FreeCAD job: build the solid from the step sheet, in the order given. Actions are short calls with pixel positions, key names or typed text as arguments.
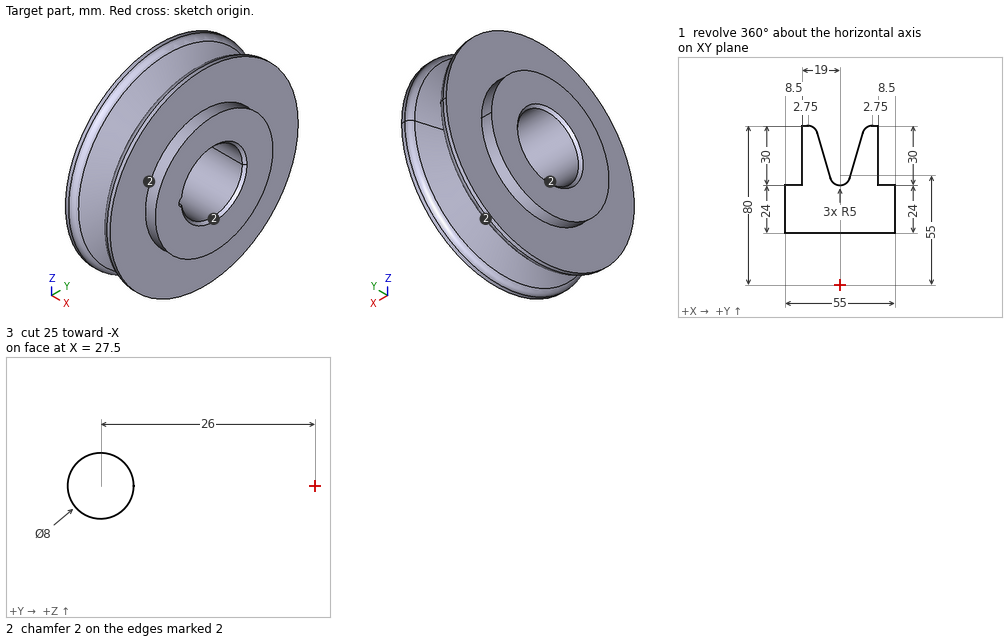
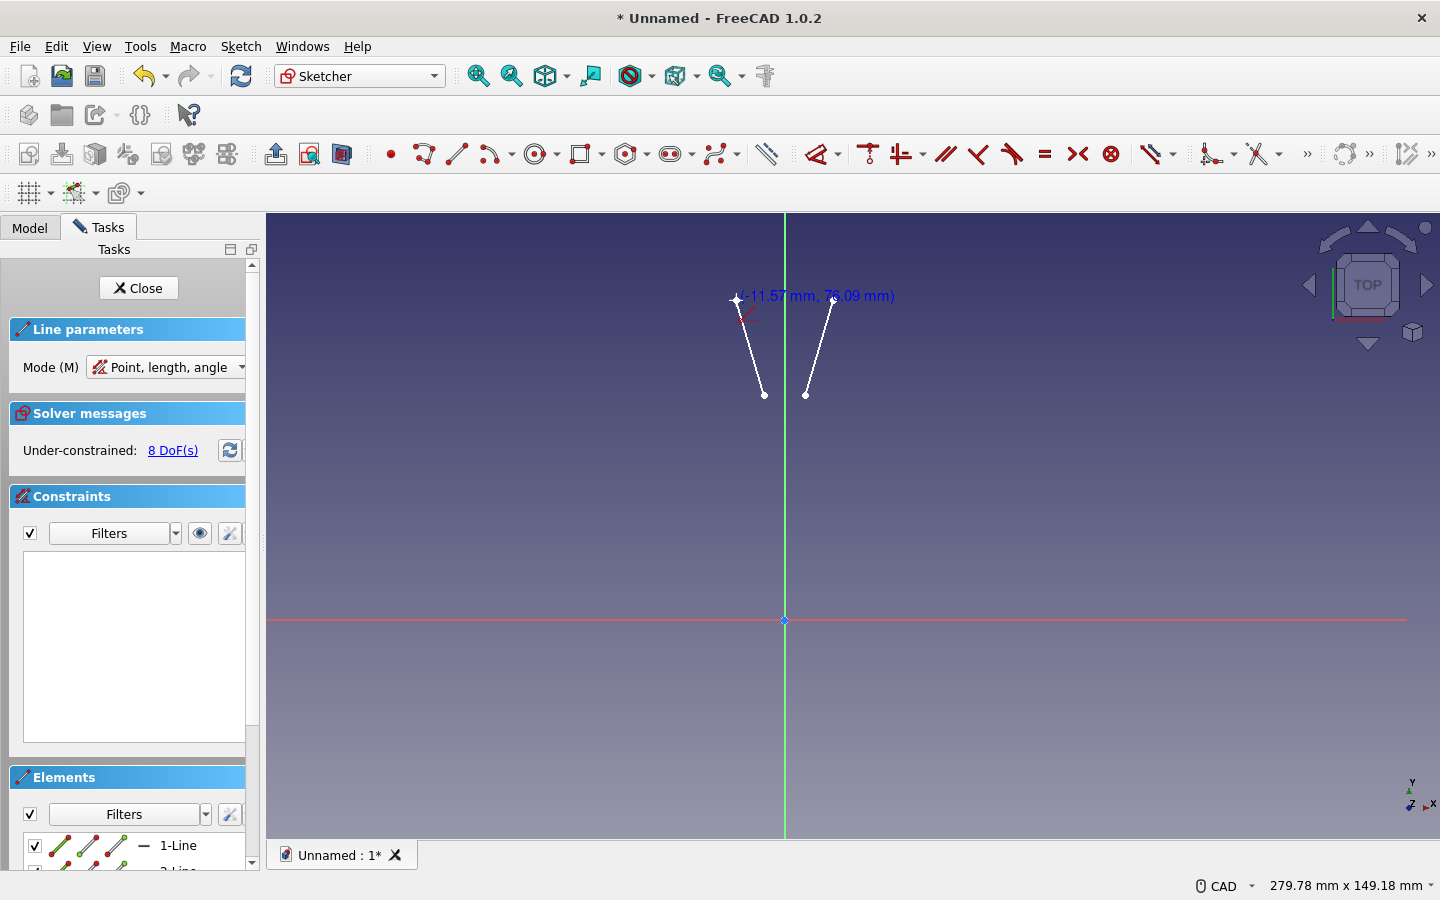
key(g)
key(m)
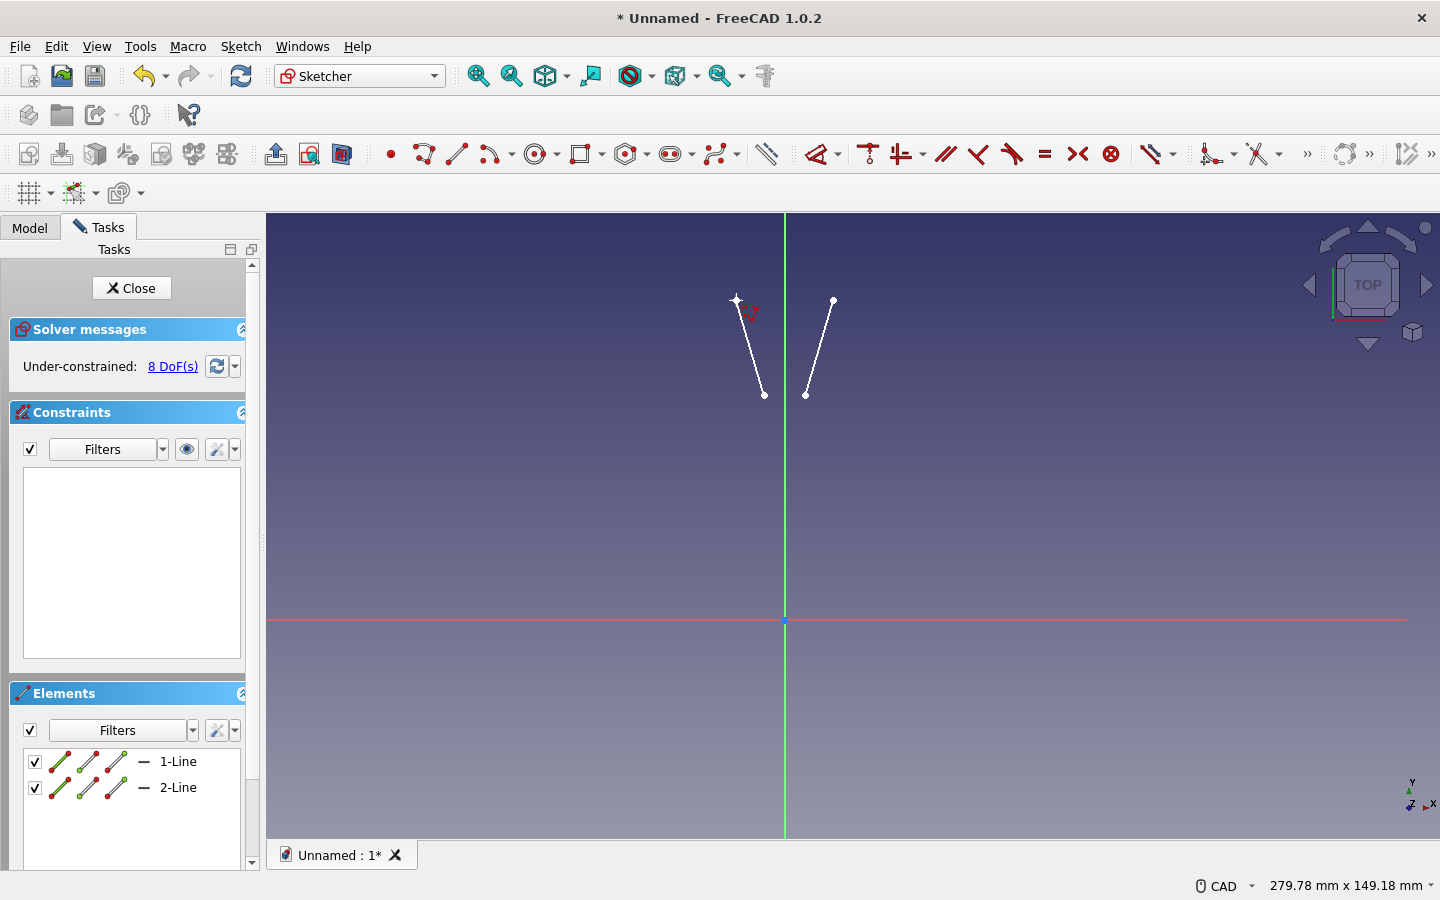
click(716, 285)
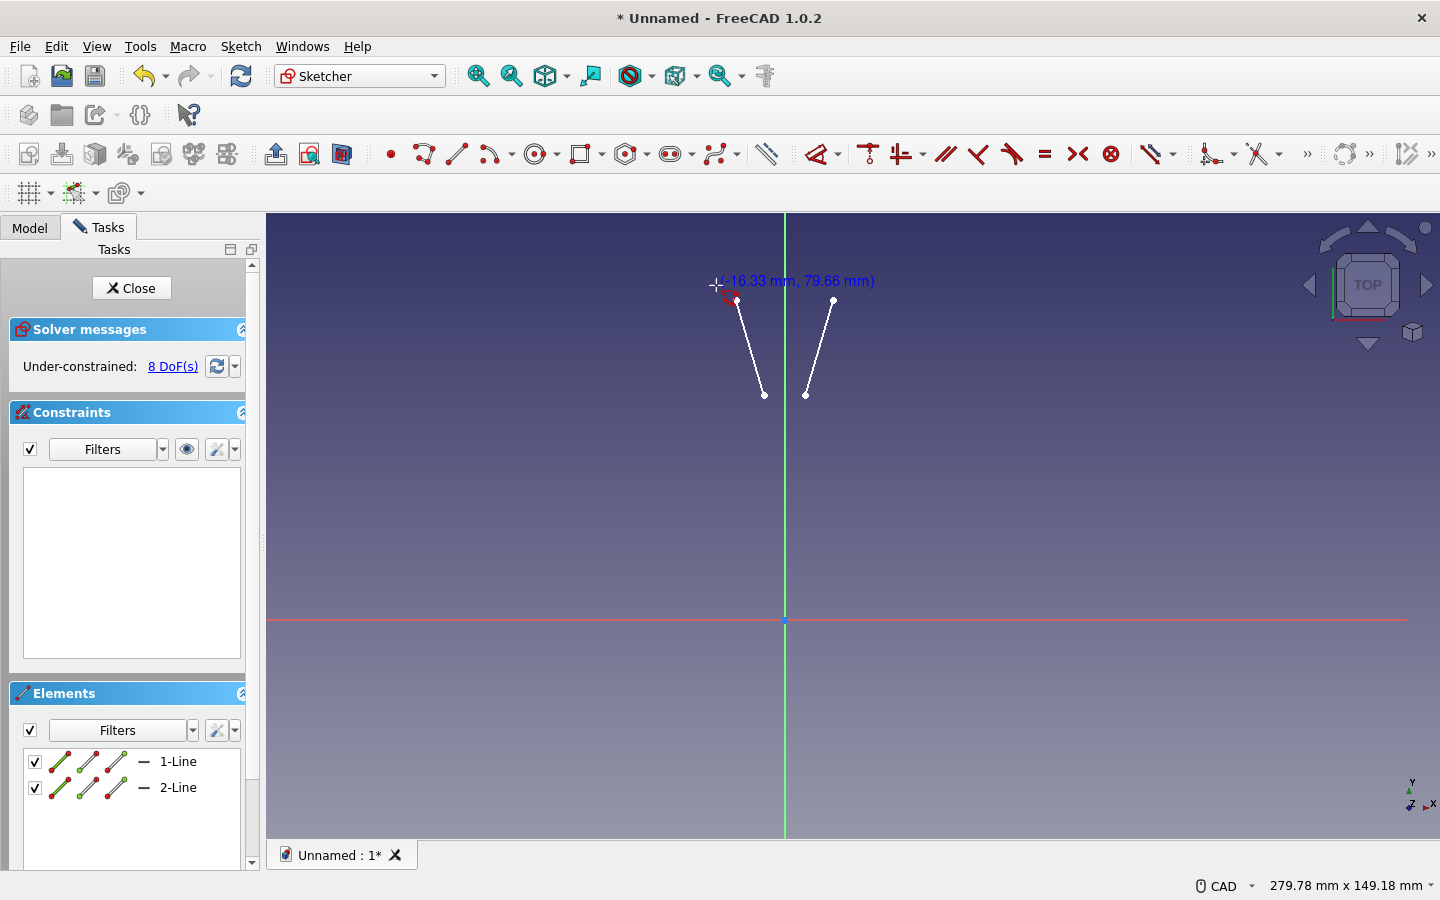
scroll(705, 285, up, 2)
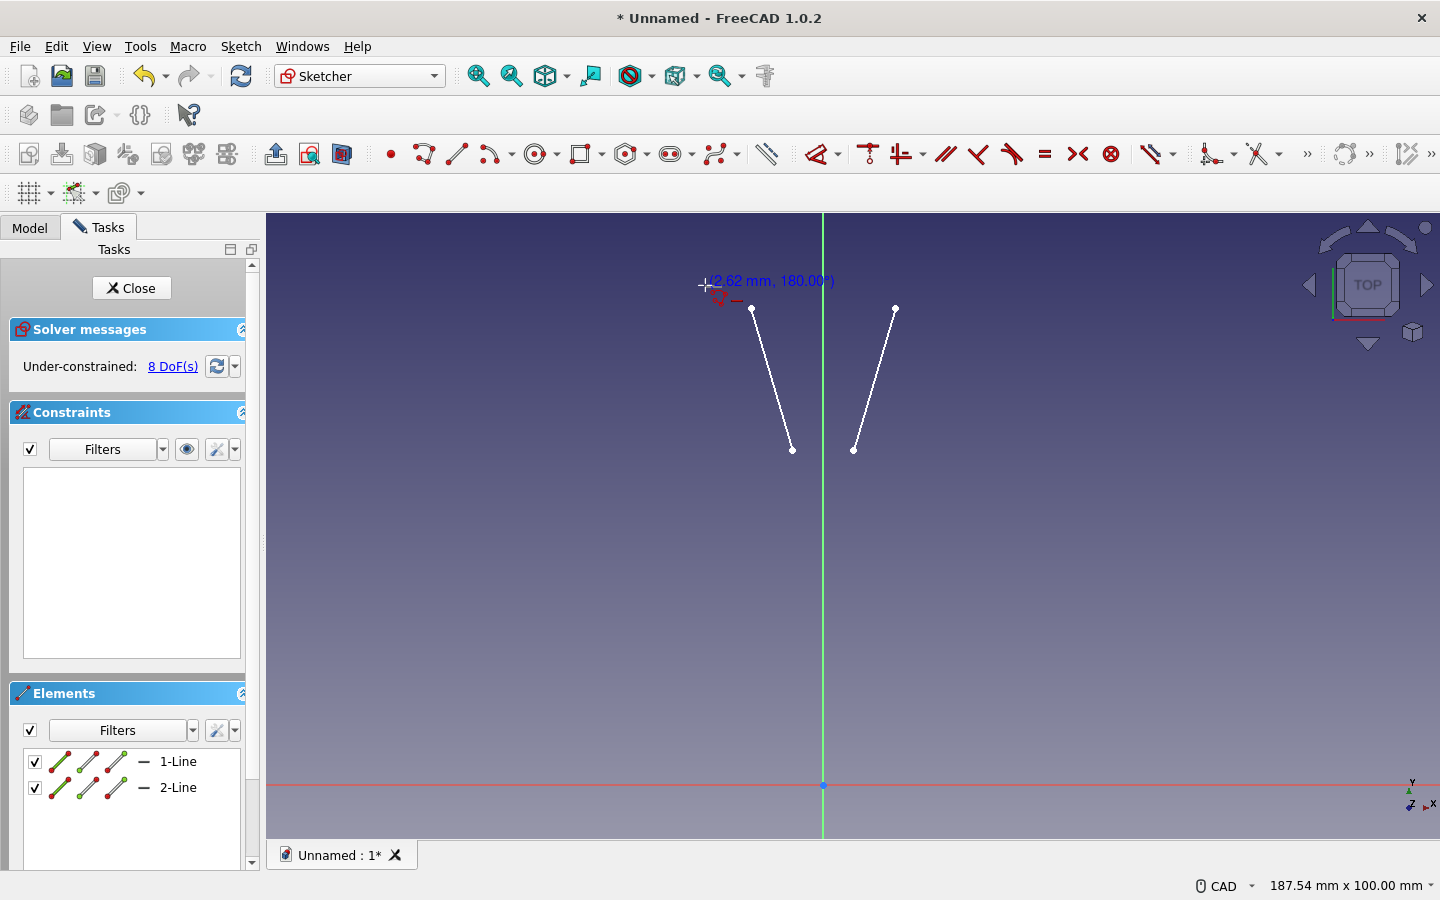
click(705, 285)
click(705, 472)
click(651, 472)
click(651, 622)
click(996, 622)
click(996, 472)
click(942, 472)
click(942, 284)
click(925, 284)
right_click(925, 284)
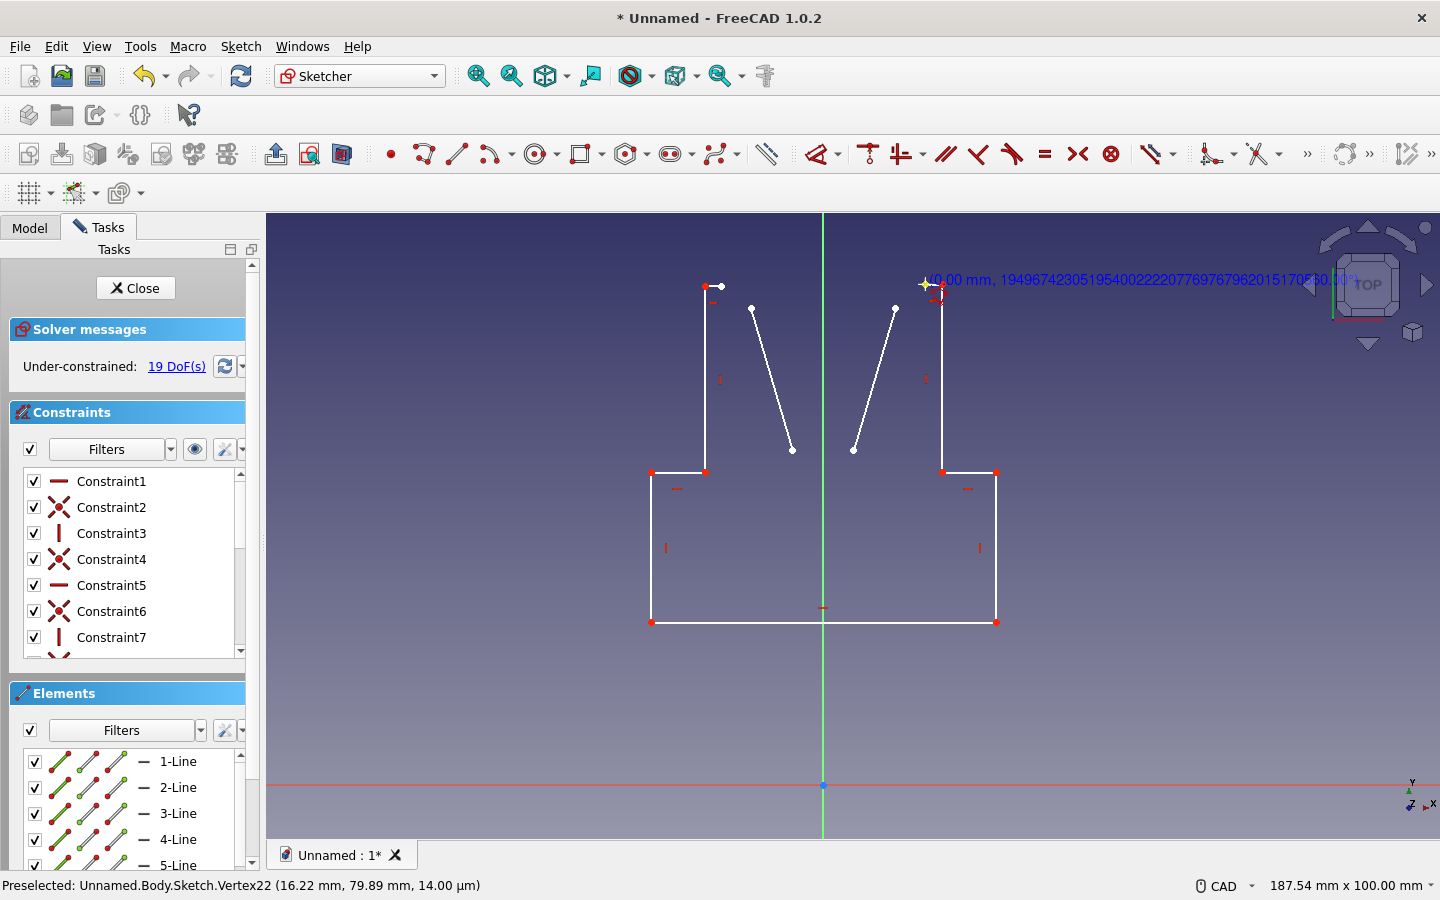
key(g)
key(3)
key(a)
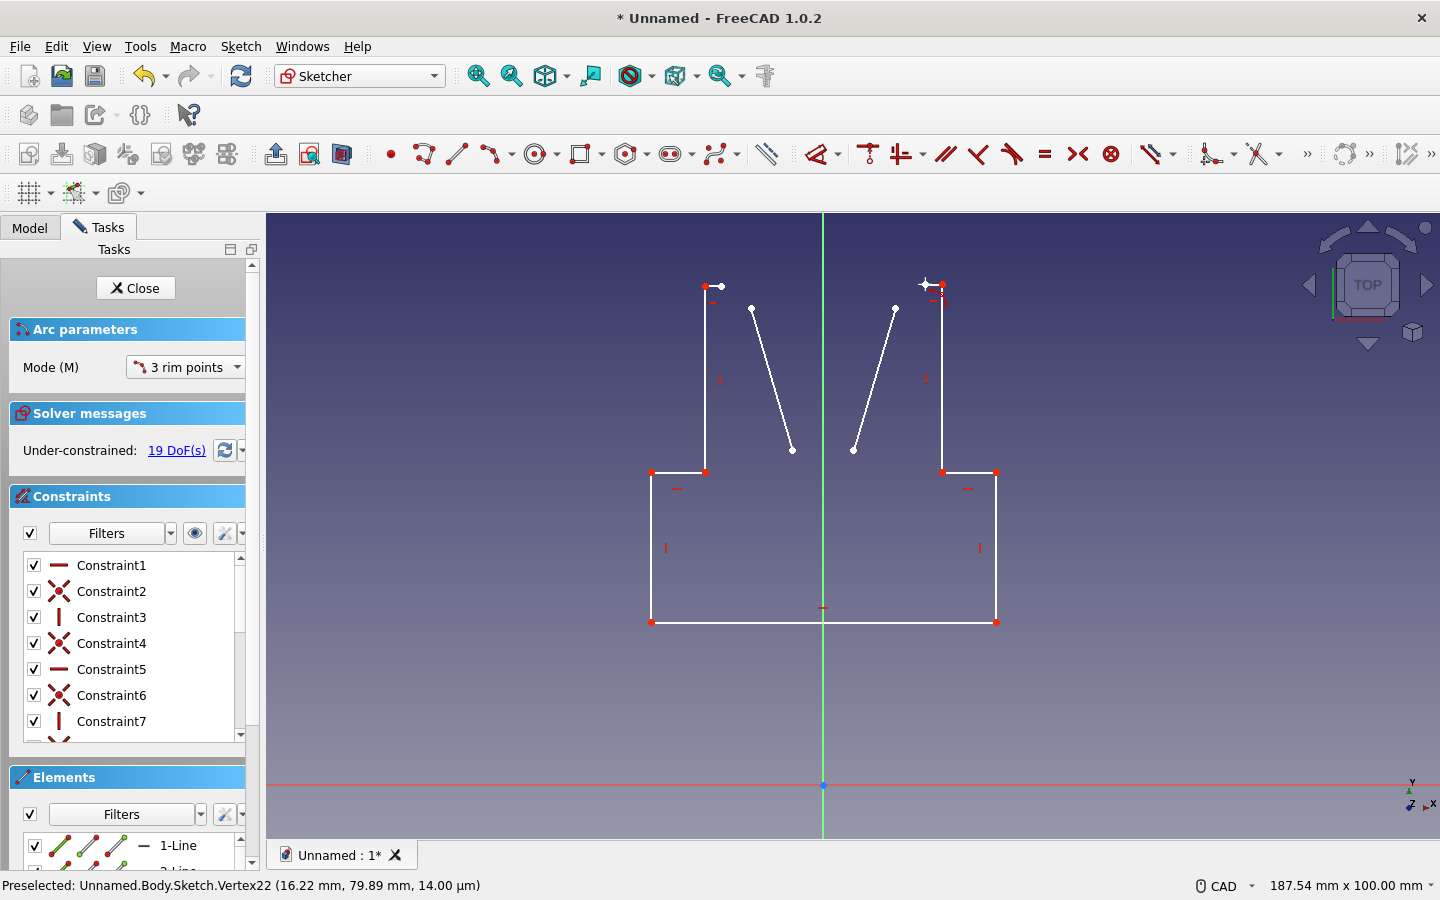
click(854, 451)
click(793, 451)
click(808, 468)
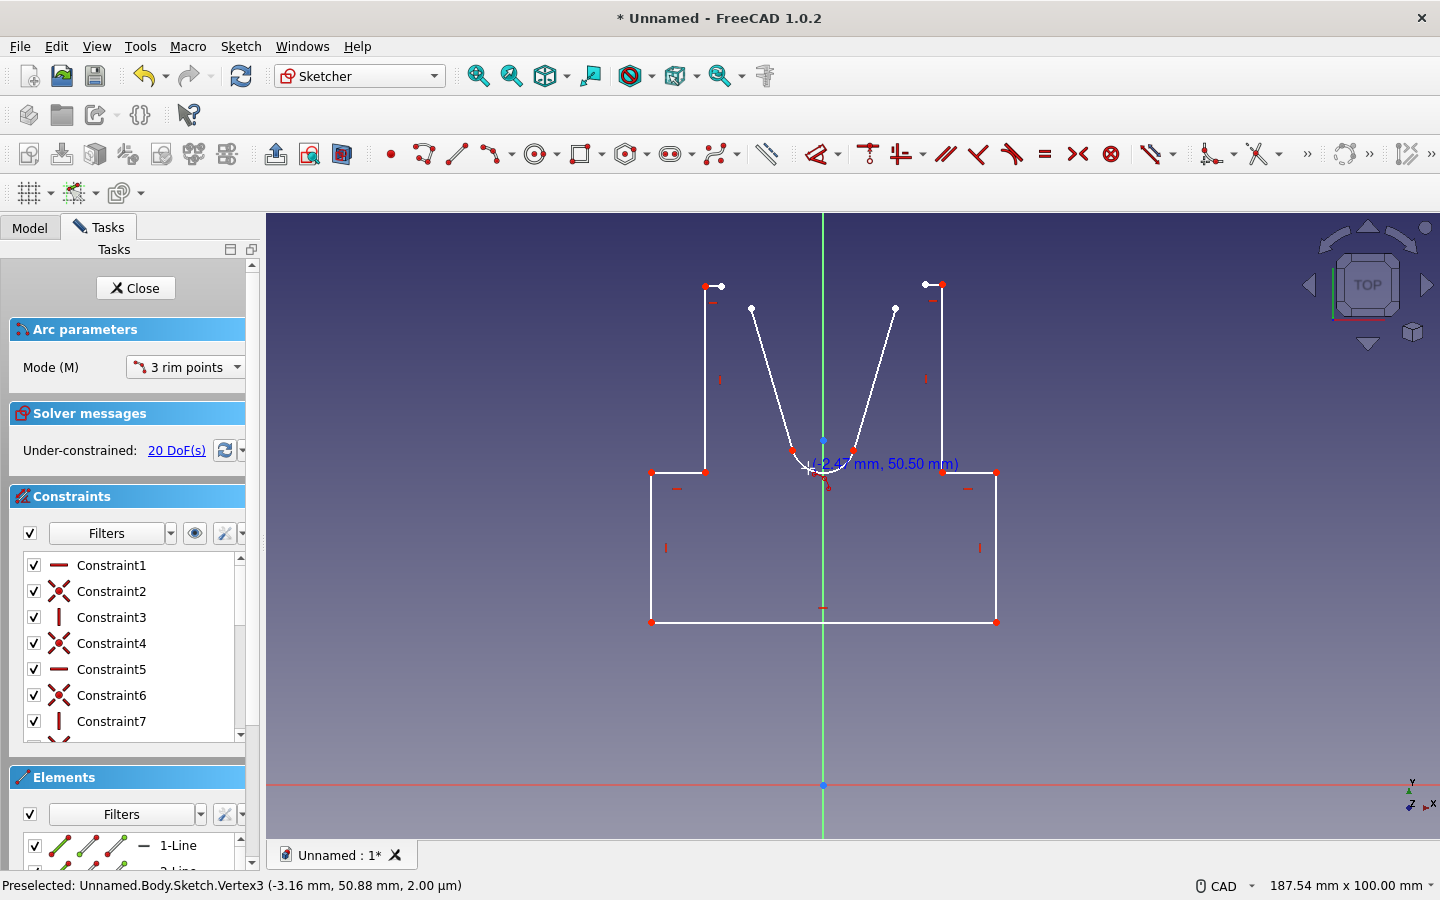
click(751, 309)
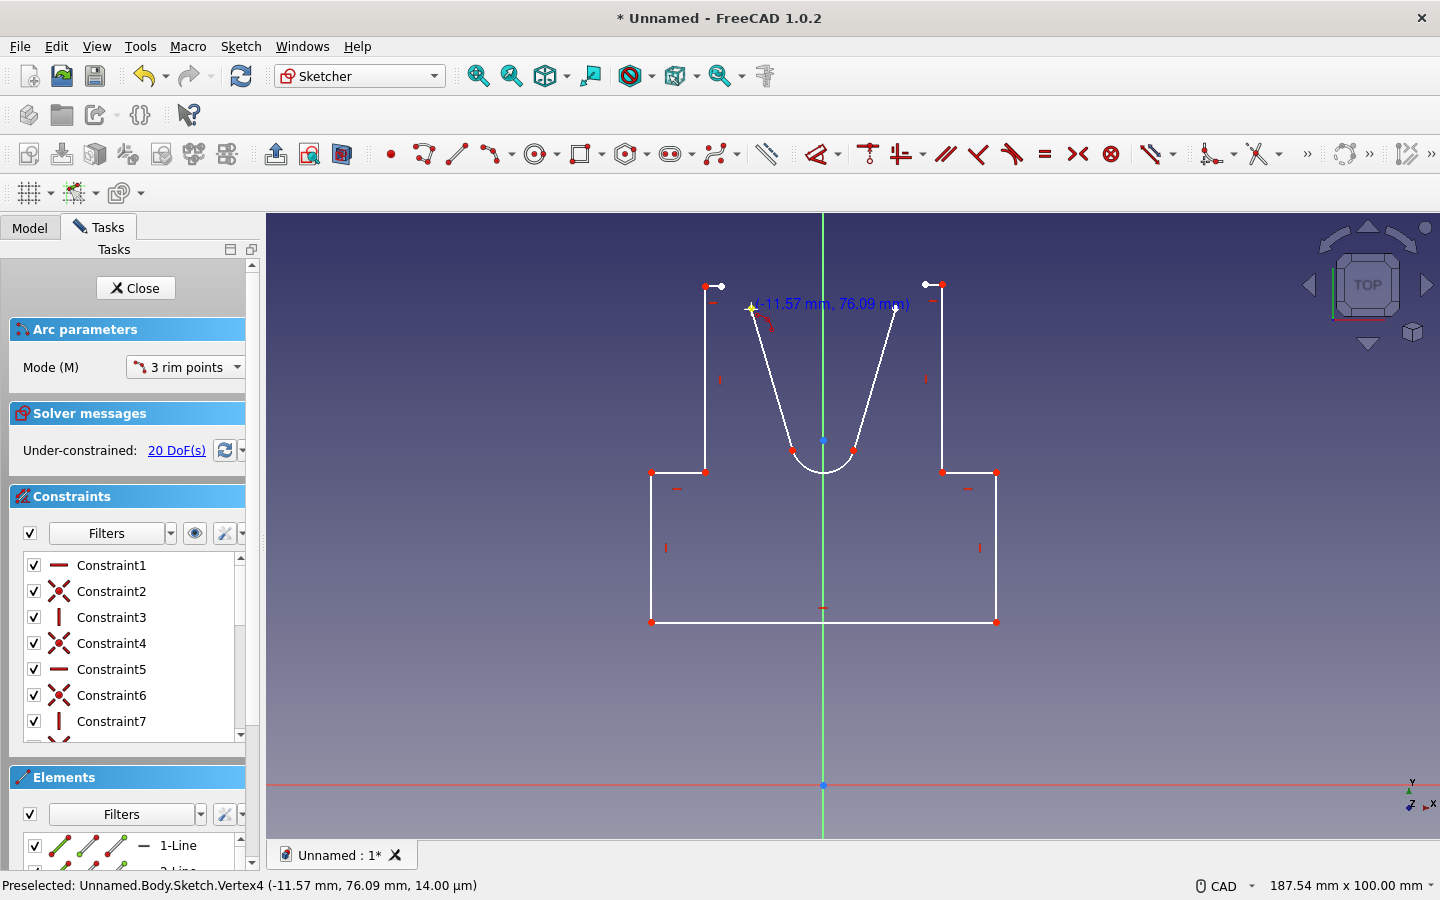
scroll(722, 284, up, 4)